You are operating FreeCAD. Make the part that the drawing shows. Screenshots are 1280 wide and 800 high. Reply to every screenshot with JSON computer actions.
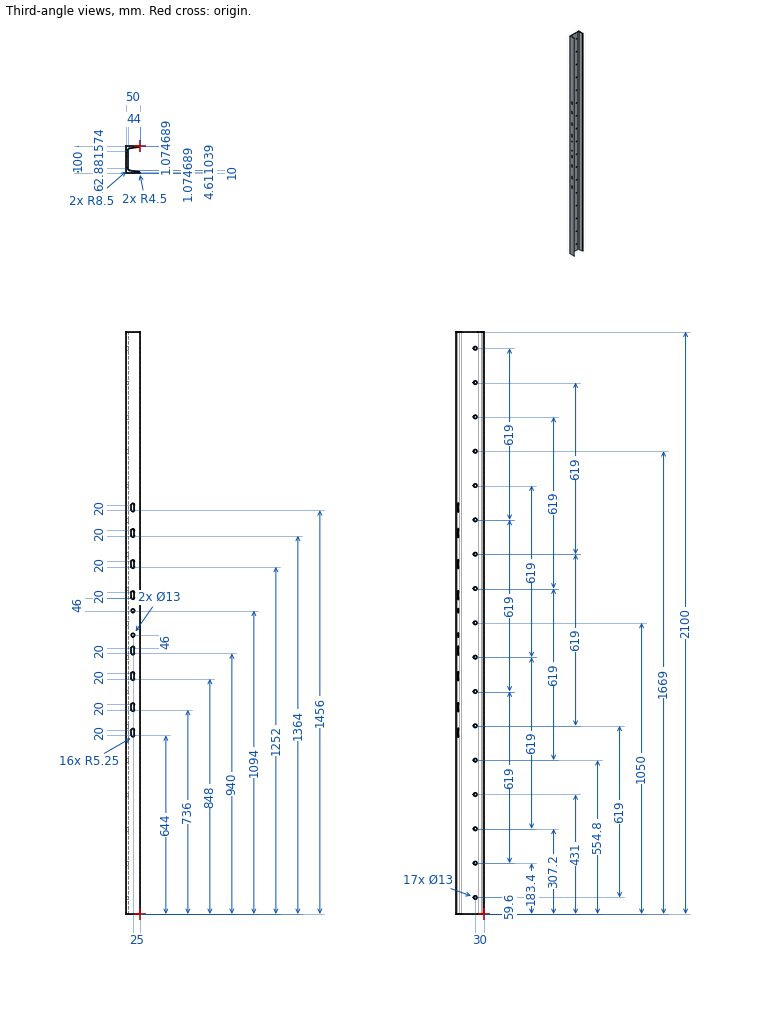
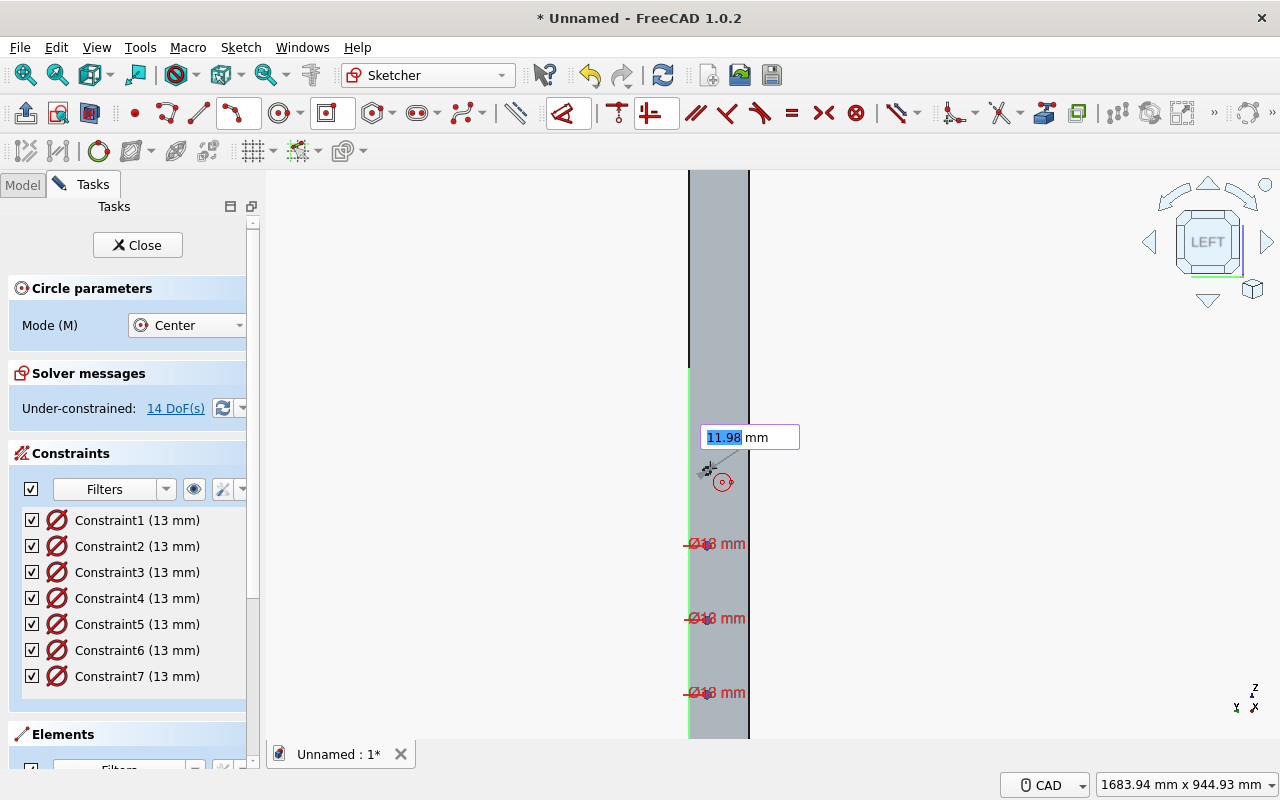
{"action": "type", "text": "13"}
{"action": "key", "text": "Return"}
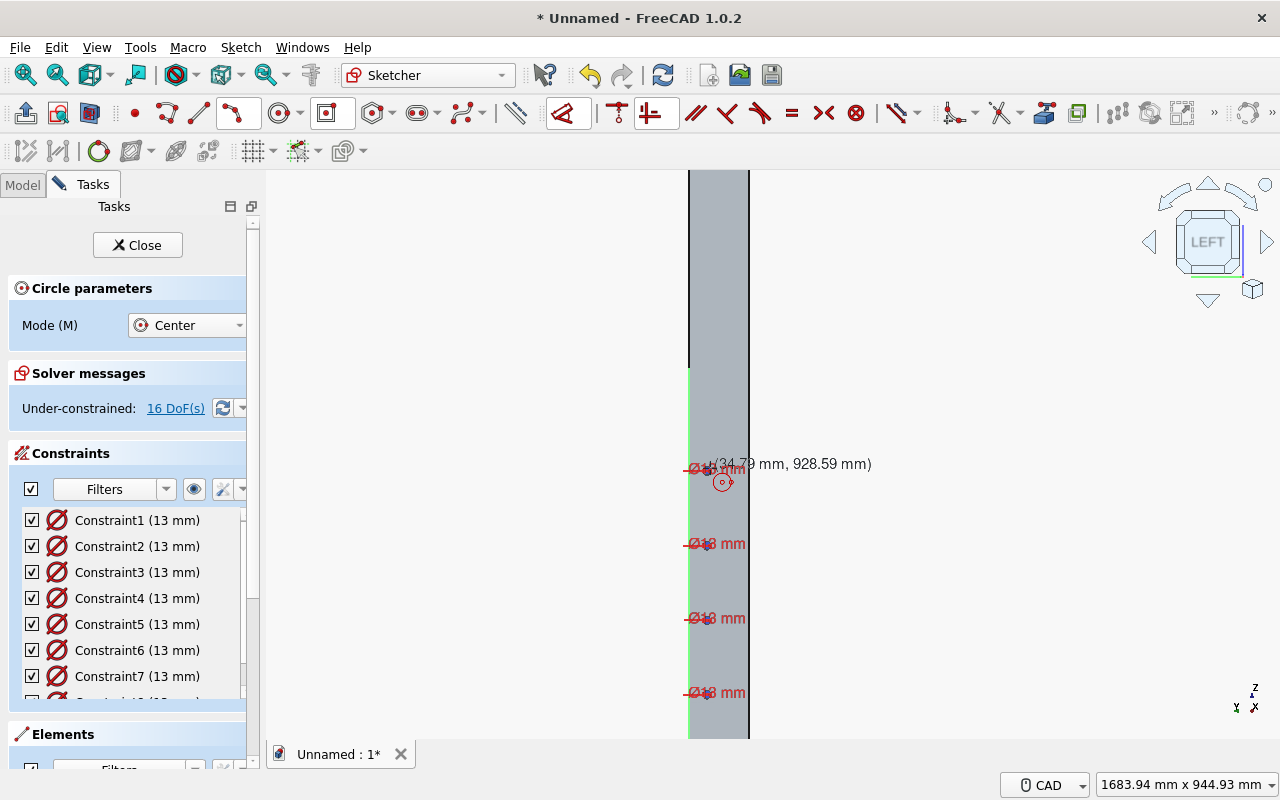
{"action": "scroll", "coordinate": [707, 396], "scroll_direction": "up", "scroll_amount": 9}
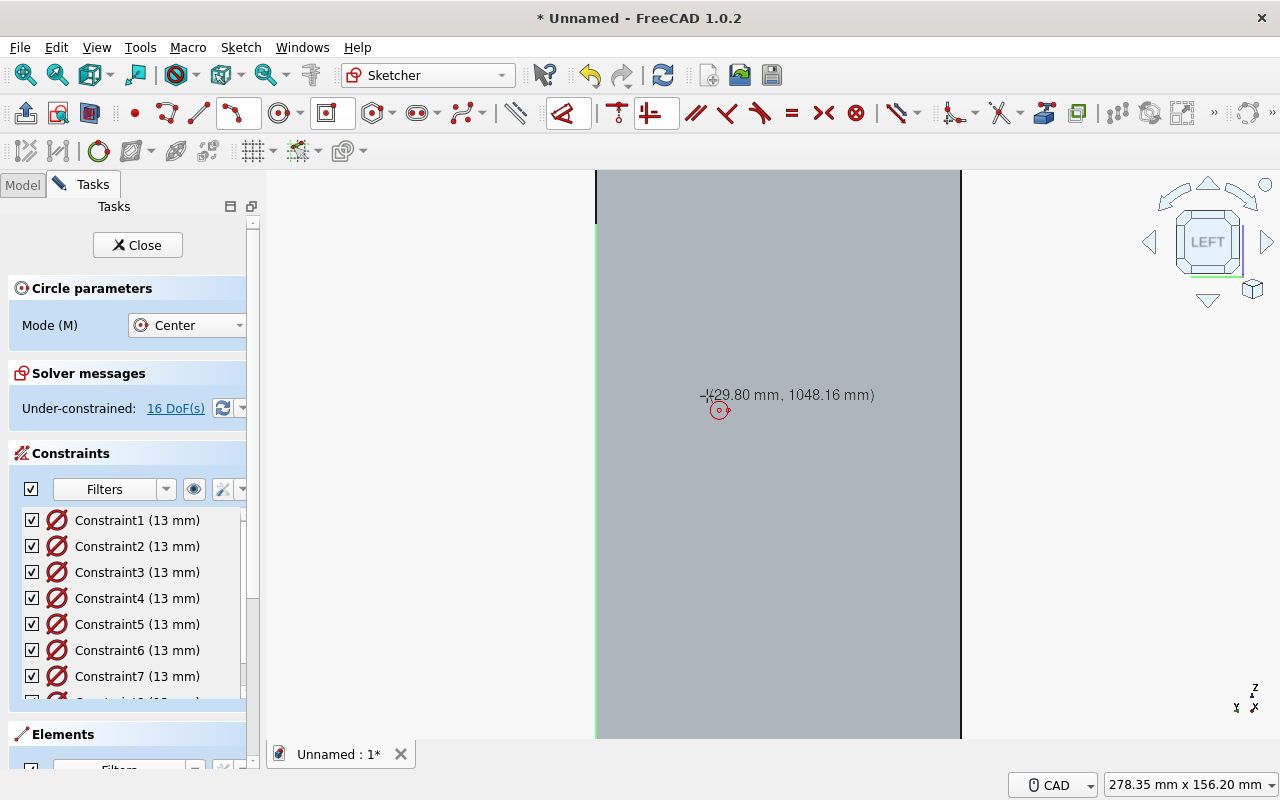
{"action": "scroll", "coordinate": [707, 453], "scroll_direction": "down", "scroll_amount": 15}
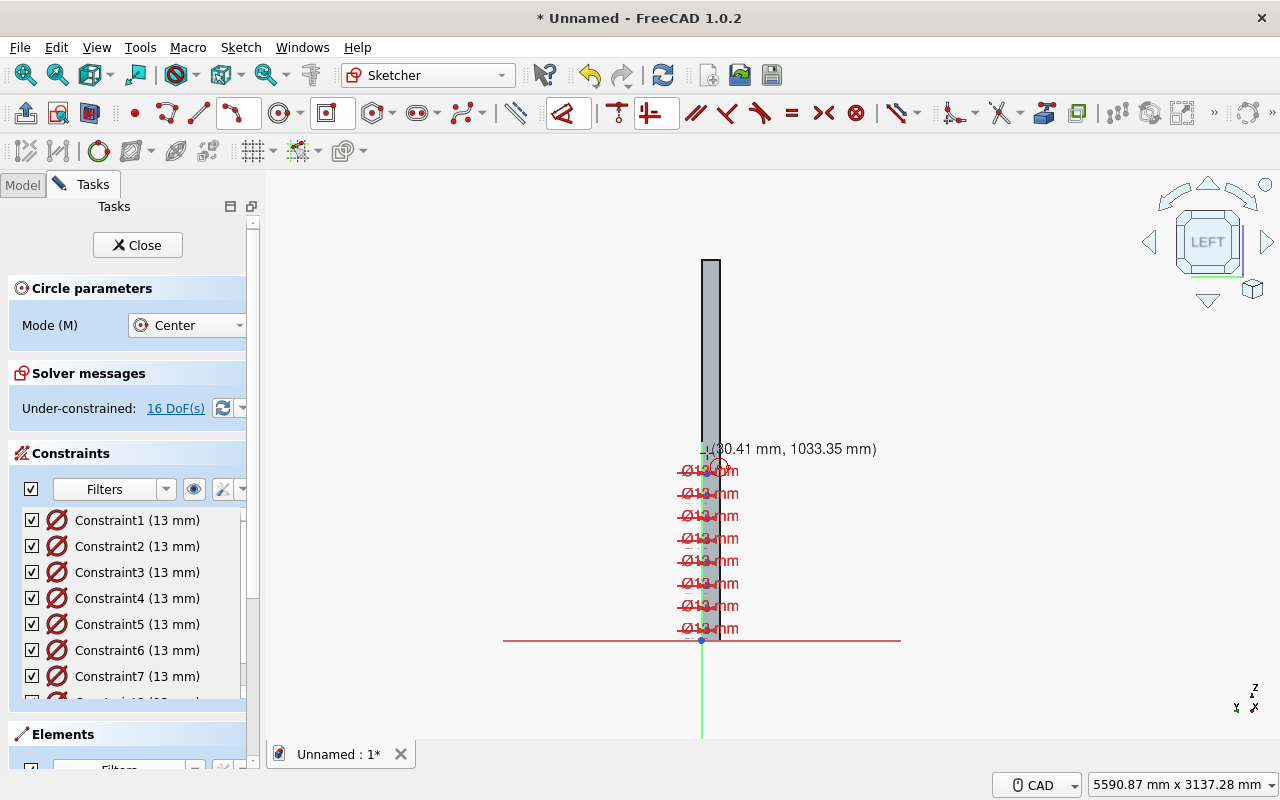
{"action": "scroll", "coordinate": [707, 451], "scroll_direction": "up", "scroll_amount": 6}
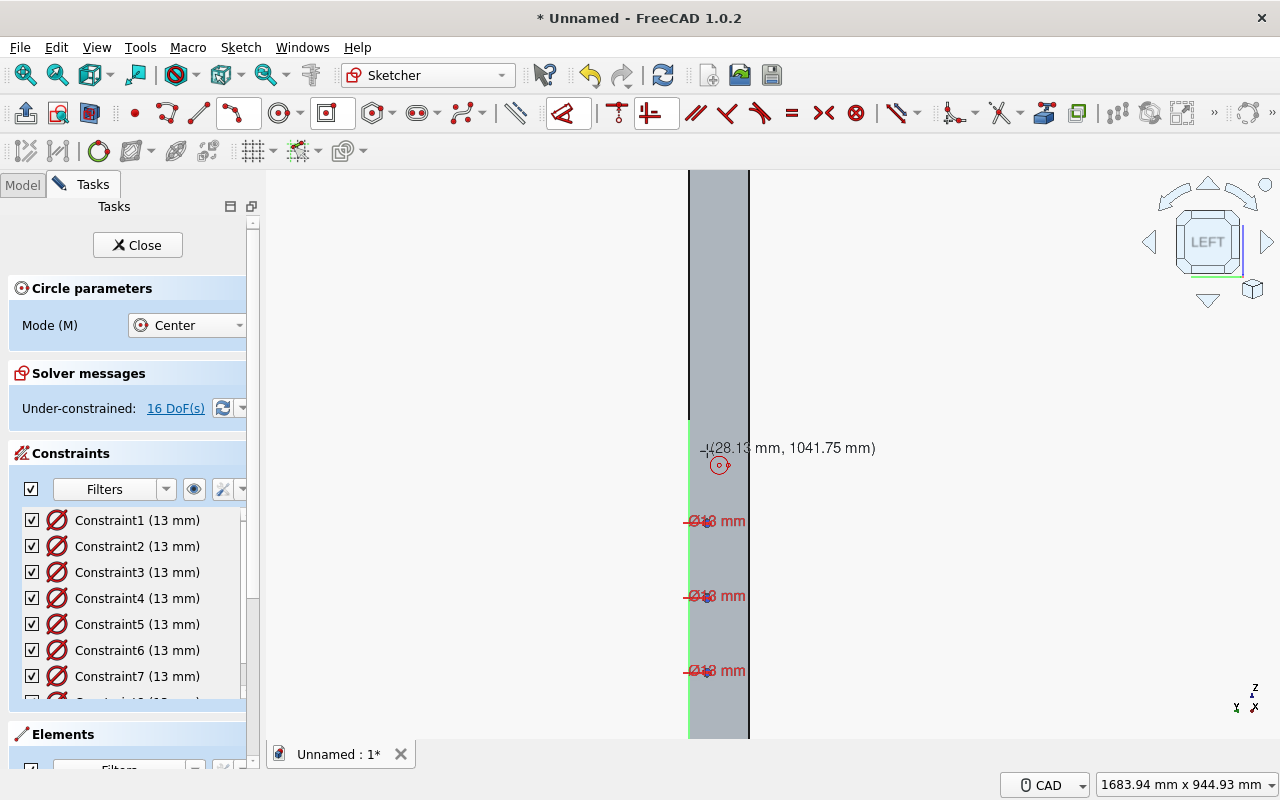
{"action": "left_click", "coordinate": [707, 448]}
{"action": "mouse_move", "coordinate": [710, 445]}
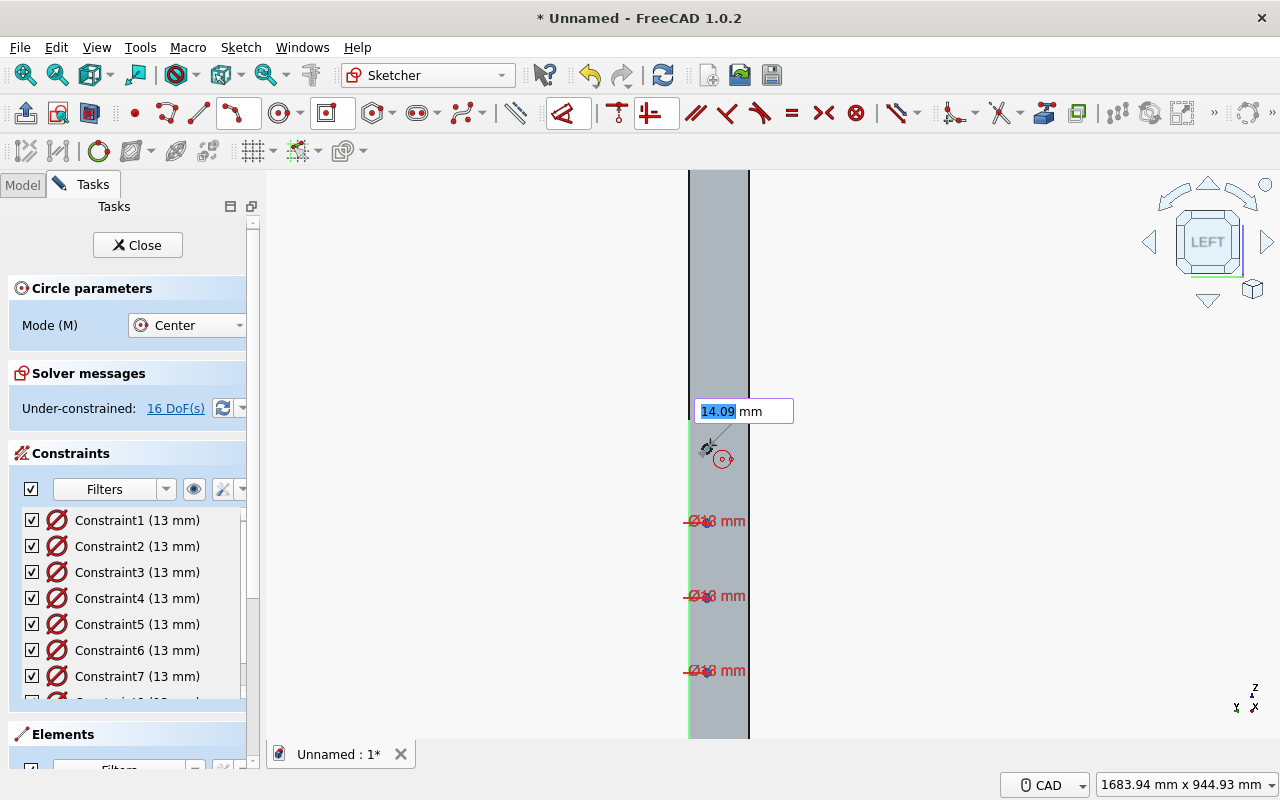
{"action": "type", "text": "13"}
{"action": "key", "text": "Return"}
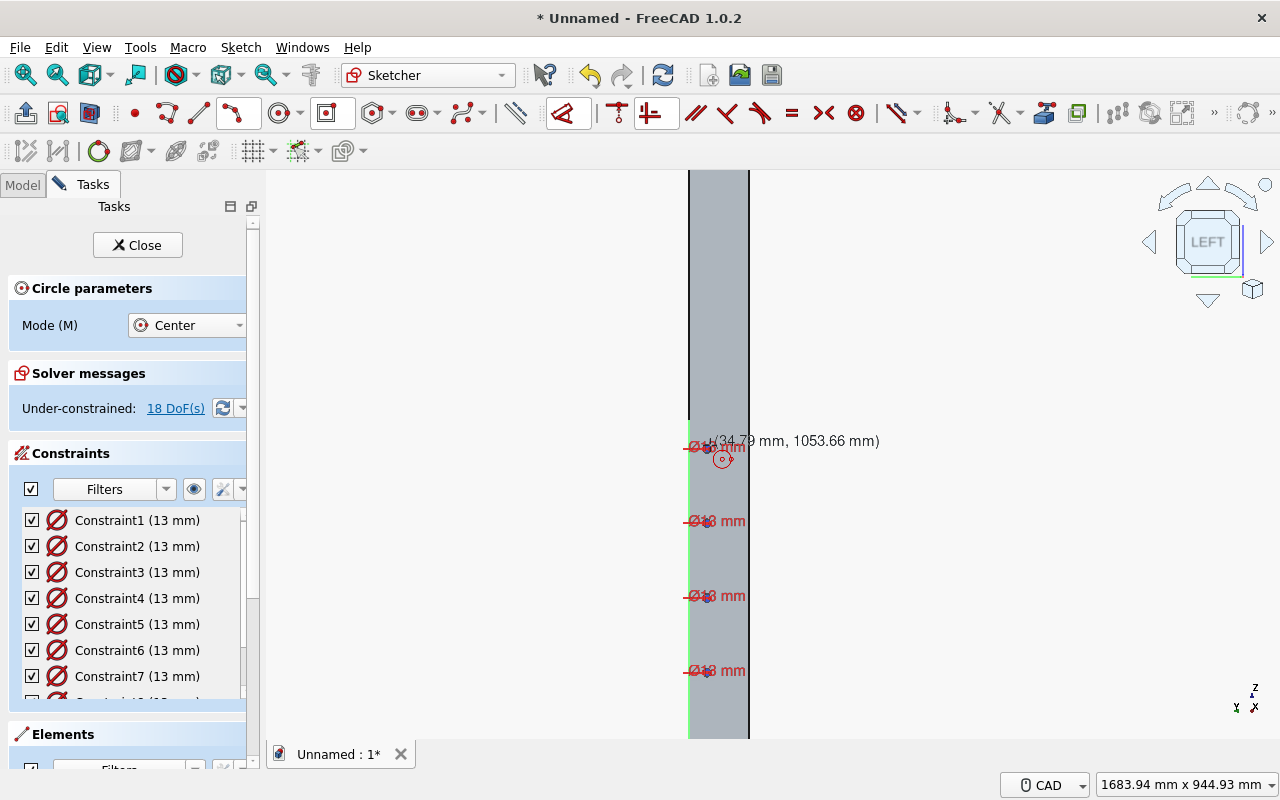
{"action": "scroll", "coordinate": [707, 374], "scroll_direction": "up", "scroll_amount": 9}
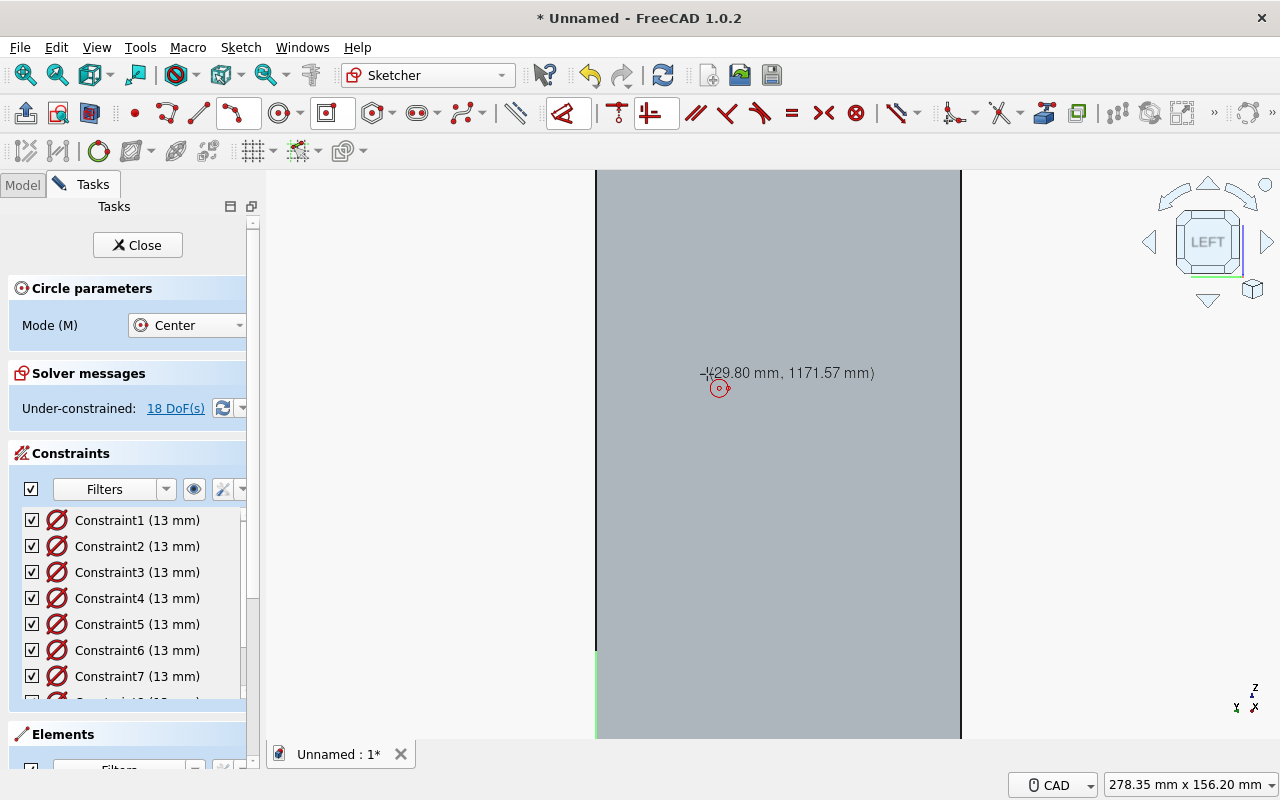
{"action": "scroll", "coordinate": [707, 430], "scroll_direction": "down", "scroll_amount": 15}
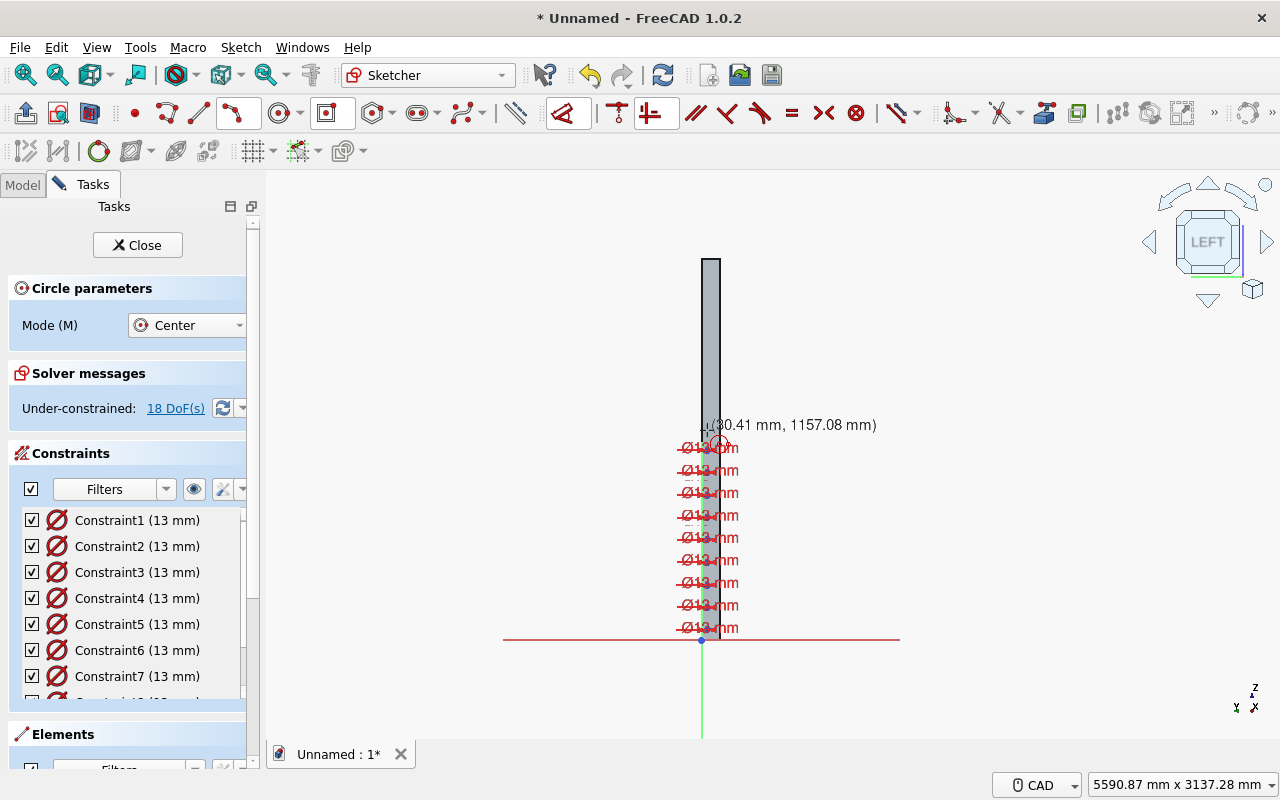
{"action": "scroll", "coordinate": [707, 427], "scroll_direction": "up", "scroll_amount": 6}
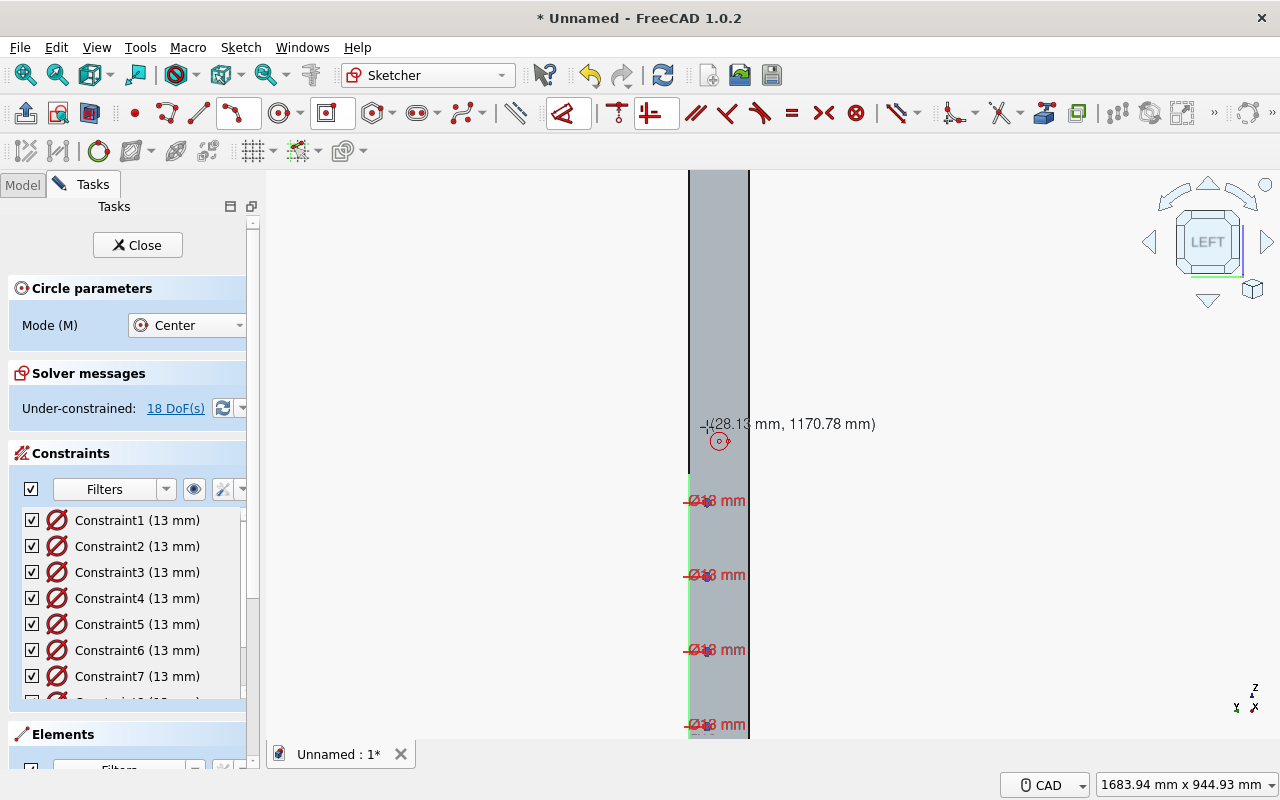
{"action": "left_click", "coordinate": [707, 427]}
{"action": "mouse_move", "coordinate": [710, 425]}